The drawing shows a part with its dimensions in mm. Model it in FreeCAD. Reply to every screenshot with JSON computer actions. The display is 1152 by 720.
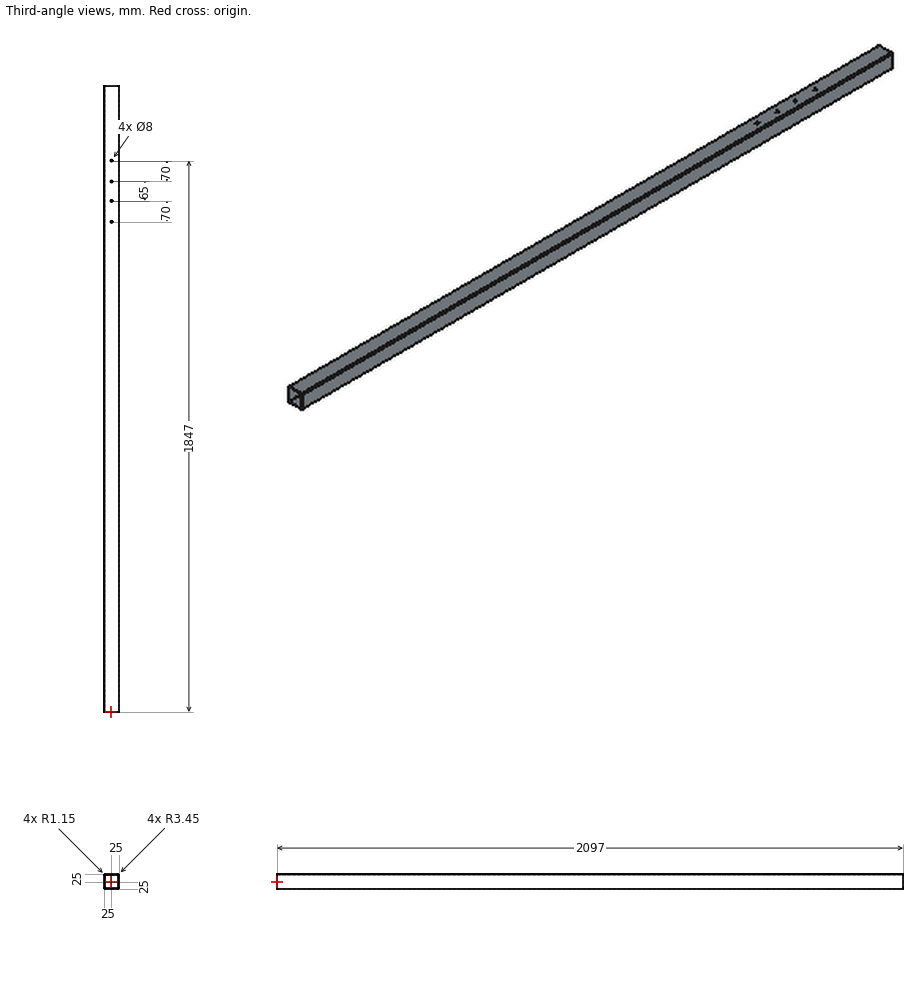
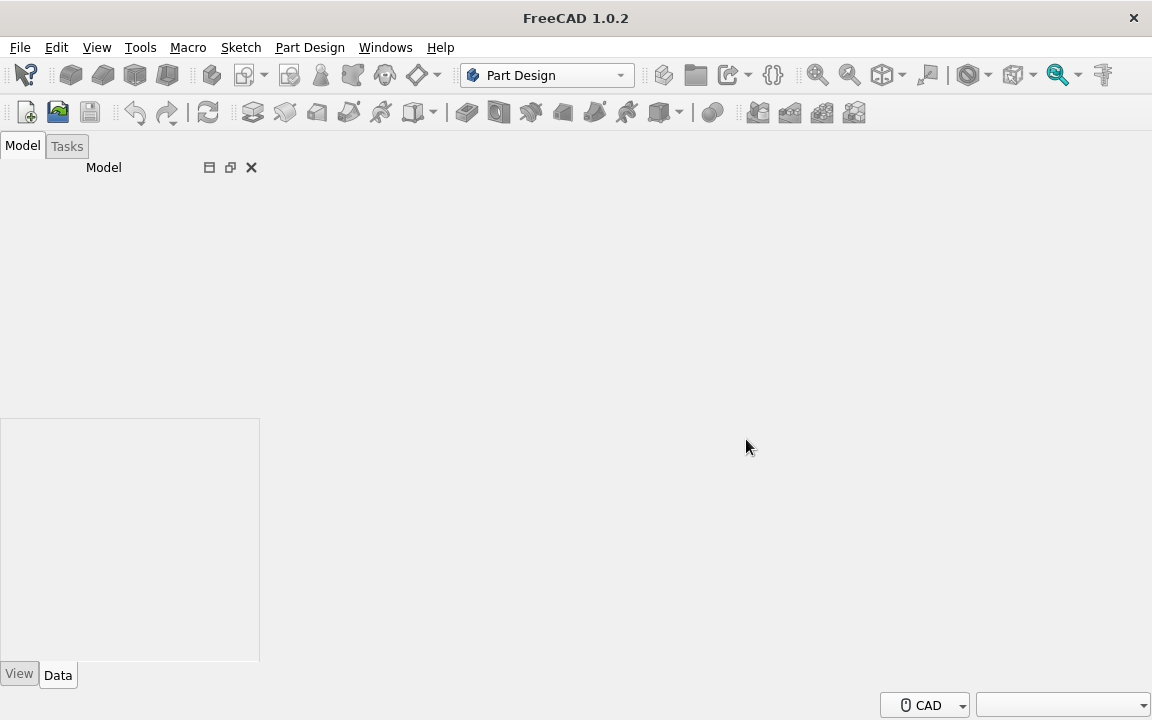
{"action": "left_click", "coordinate": [26, 112]}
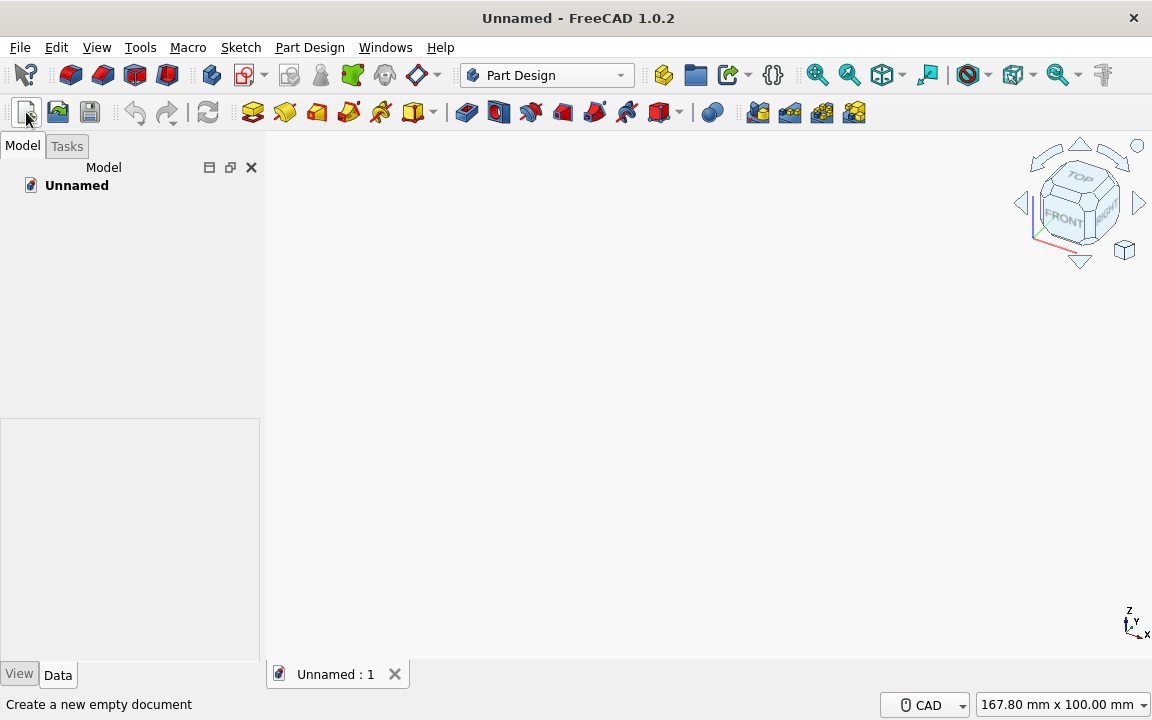
{"action": "left_click", "coordinate": [244, 76]}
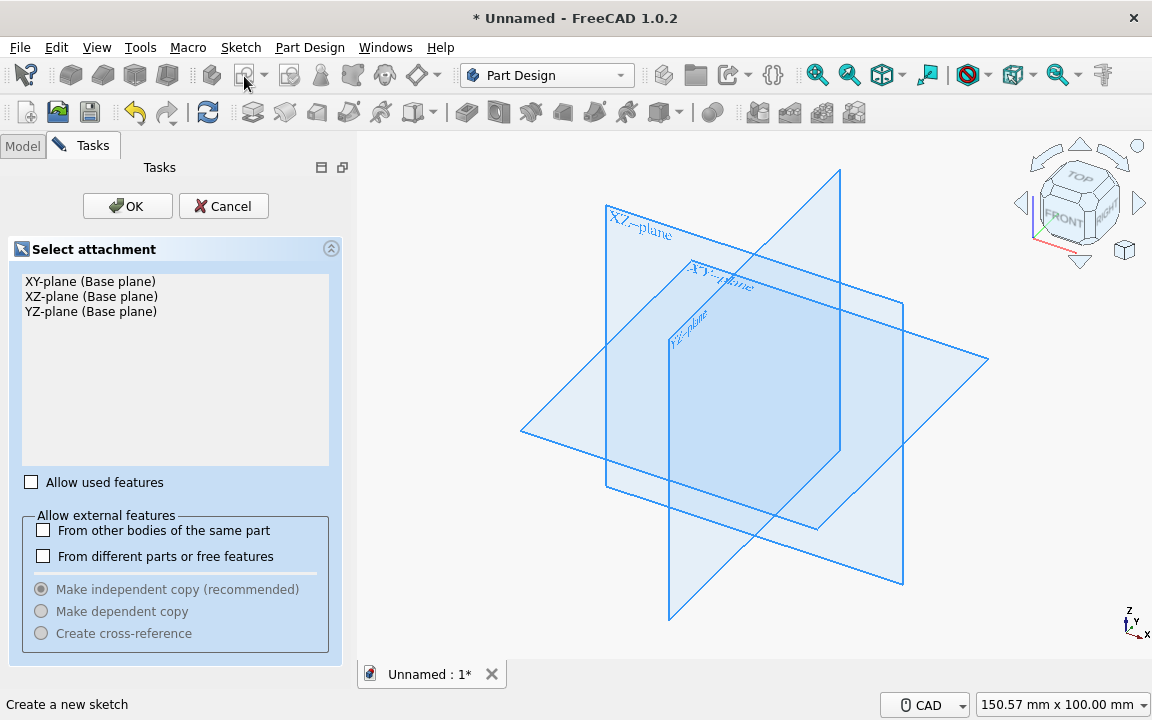
{"action": "left_click", "coordinate": [82, 296]}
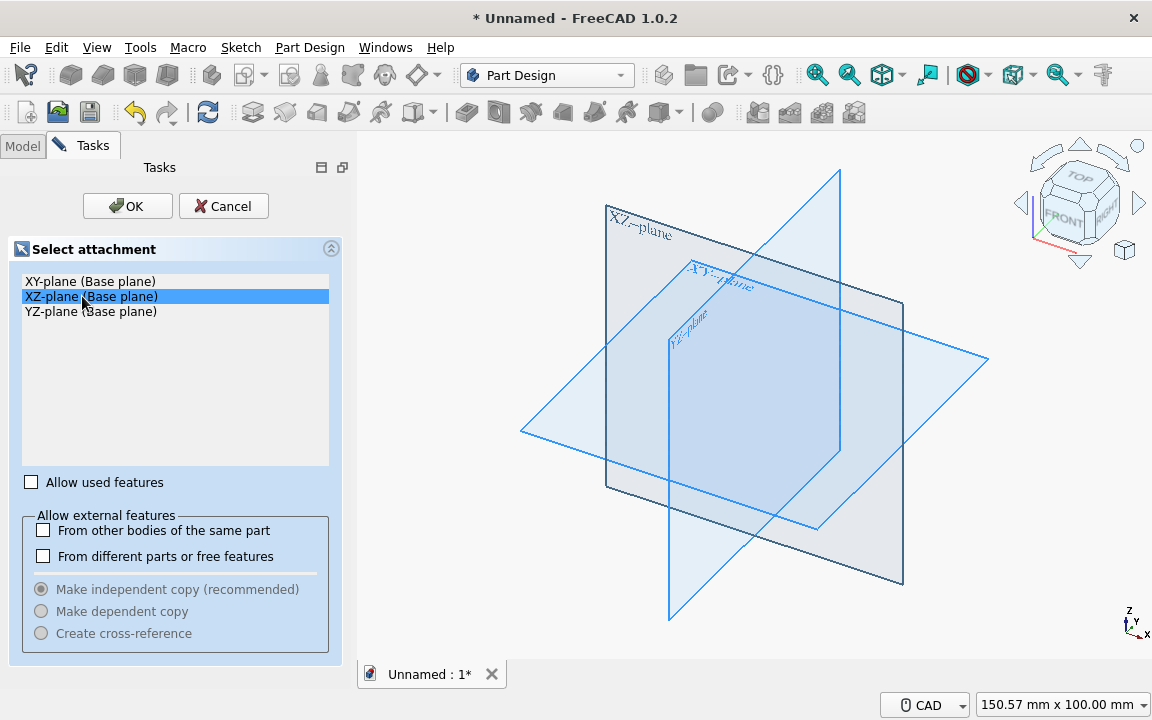
{"action": "left_click", "coordinate": [128, 206]}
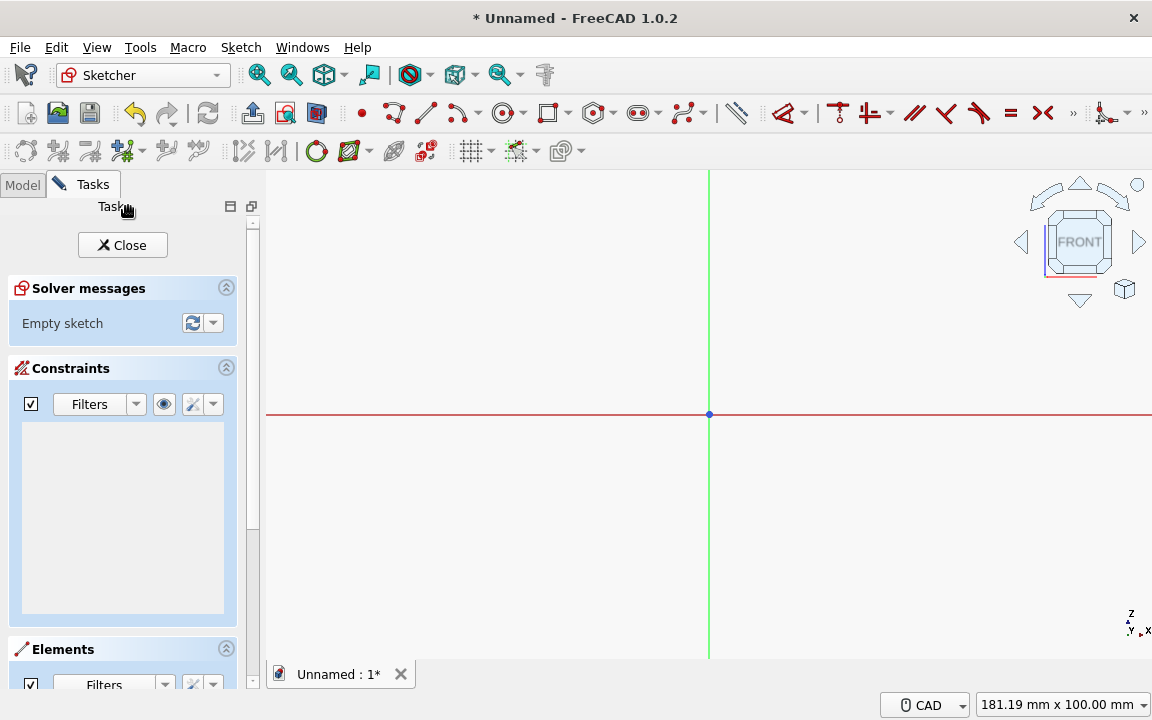
{"action": "left_click", "coordinate": [426, 114]}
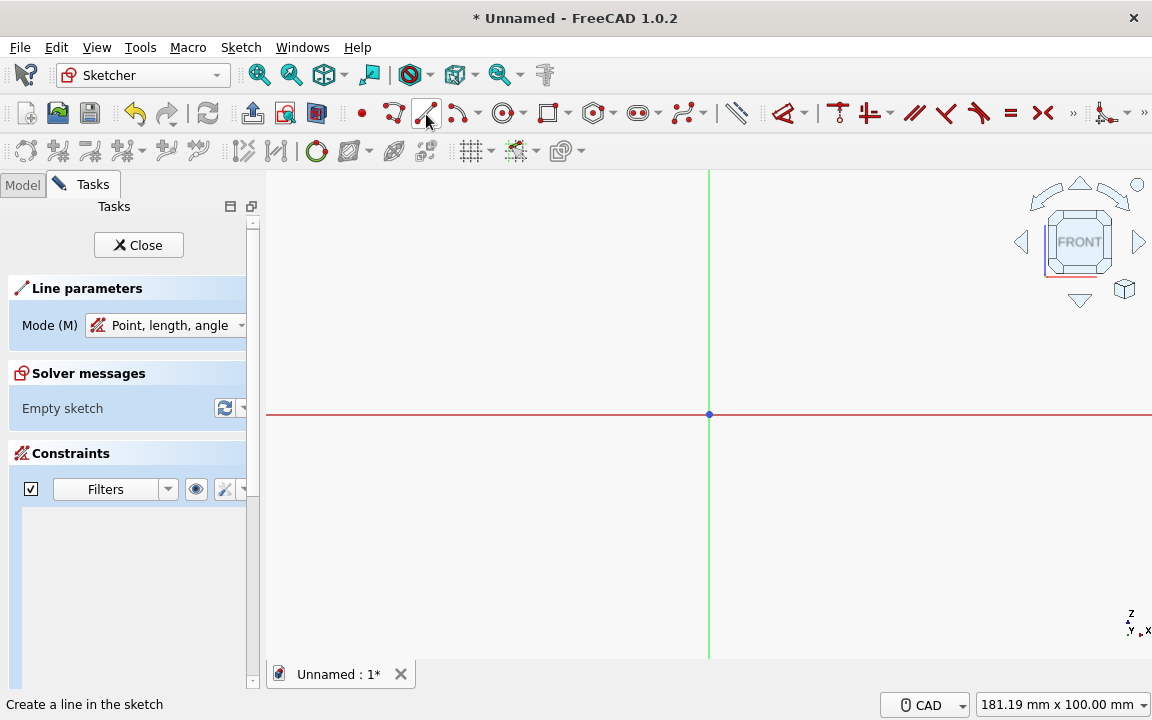
{"action": "left_click", "coordinate": [604, 292]}
{"action": "left_click", "coordinate": [814, 292]}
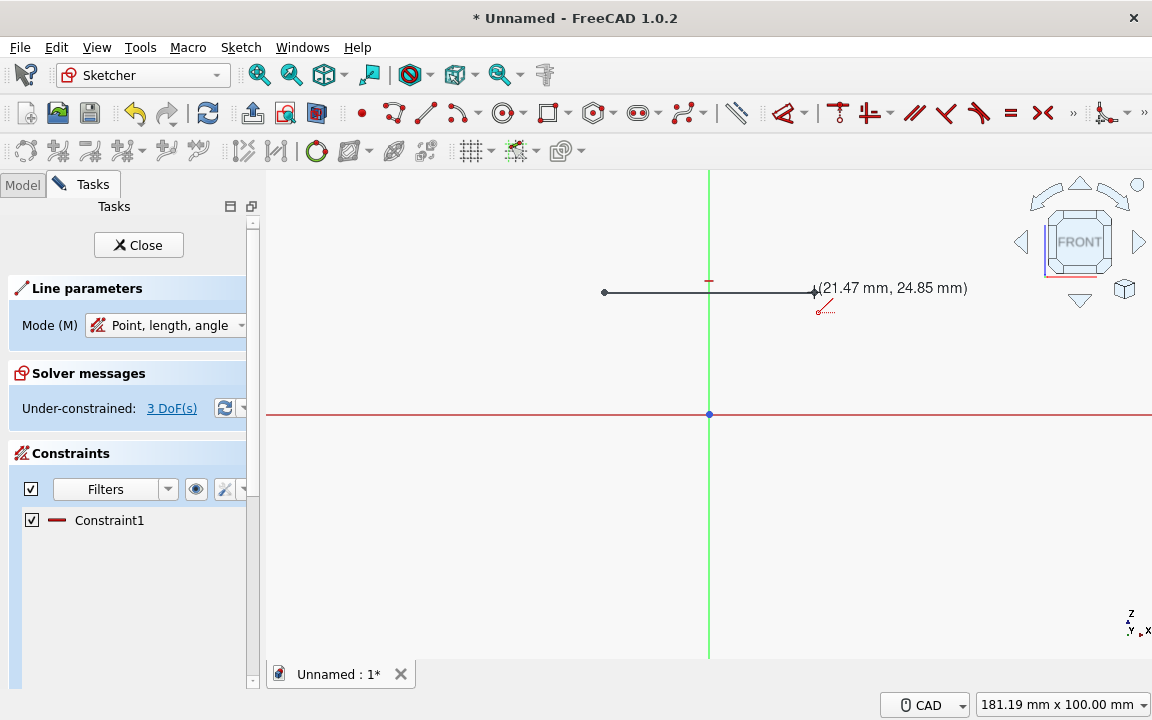
{"action": "left_click", "coordinate": [831, 309]}
{"action": "left_click", "coordinate": [831, 520]}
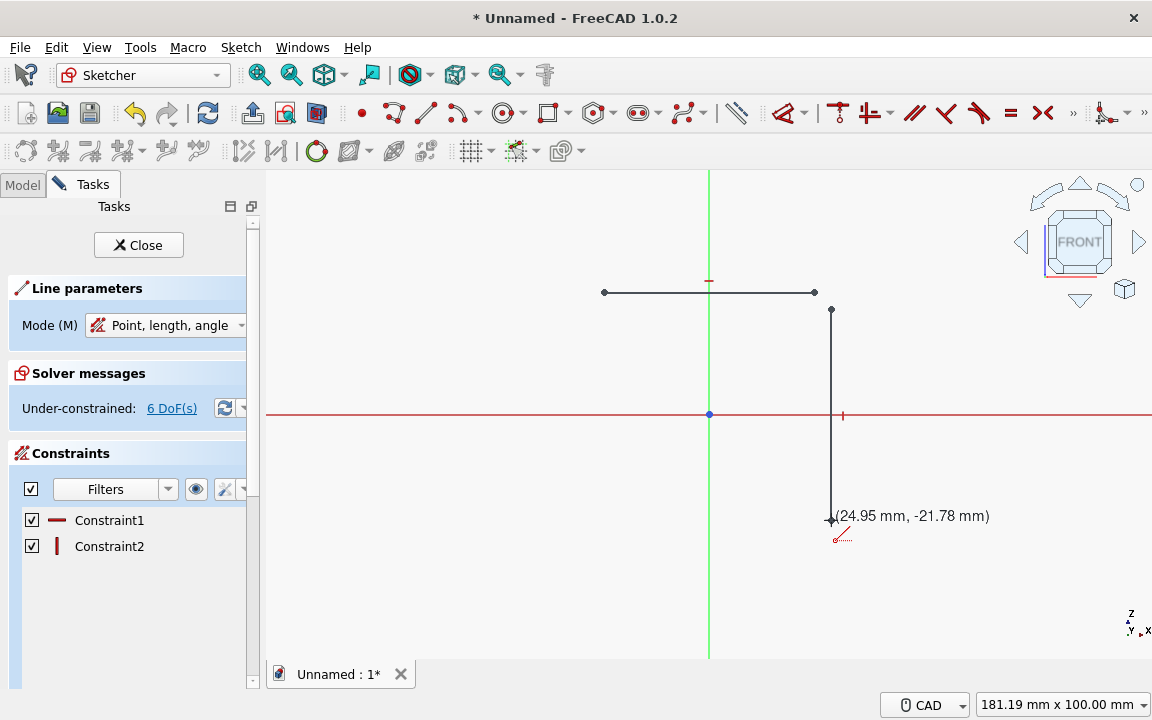
{"action": "left_click", "coordinate": [814, 537]}
{"action": "left_click", "coordinate": [604, 537]}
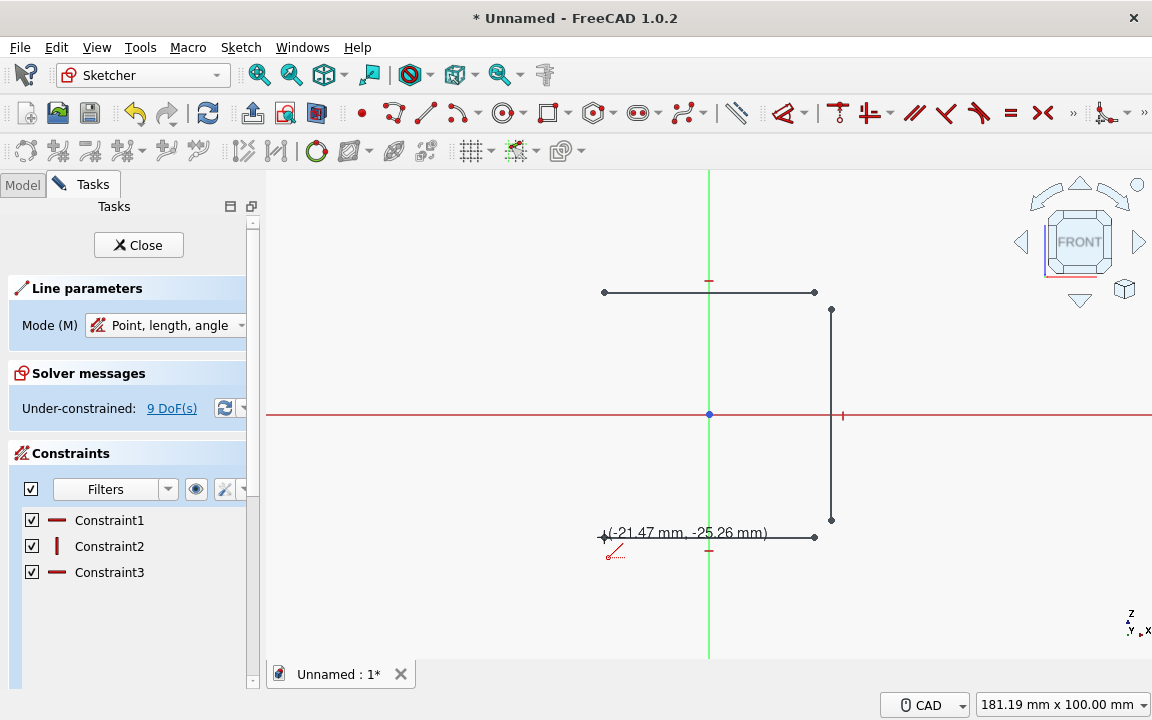
{"action": "left_click", "coordinate": [587, 520]}
{"action": "left_click", "coordinate": [587, 309]}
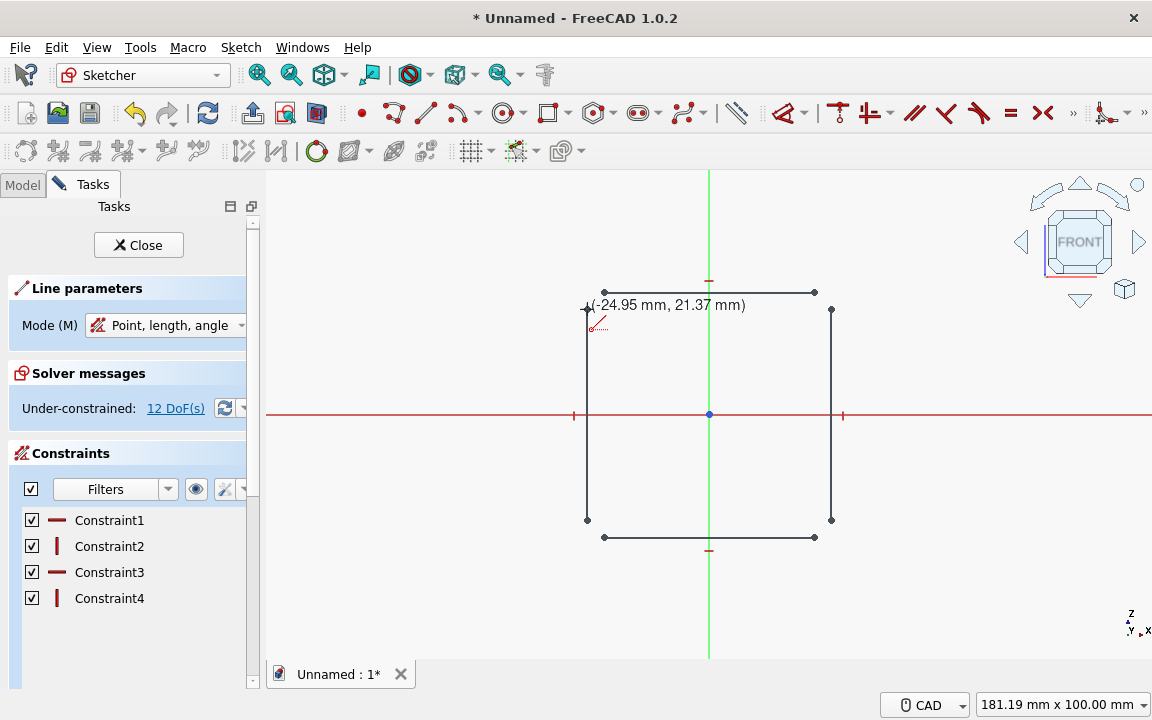
{"action": "key", "text": "g 3 a"}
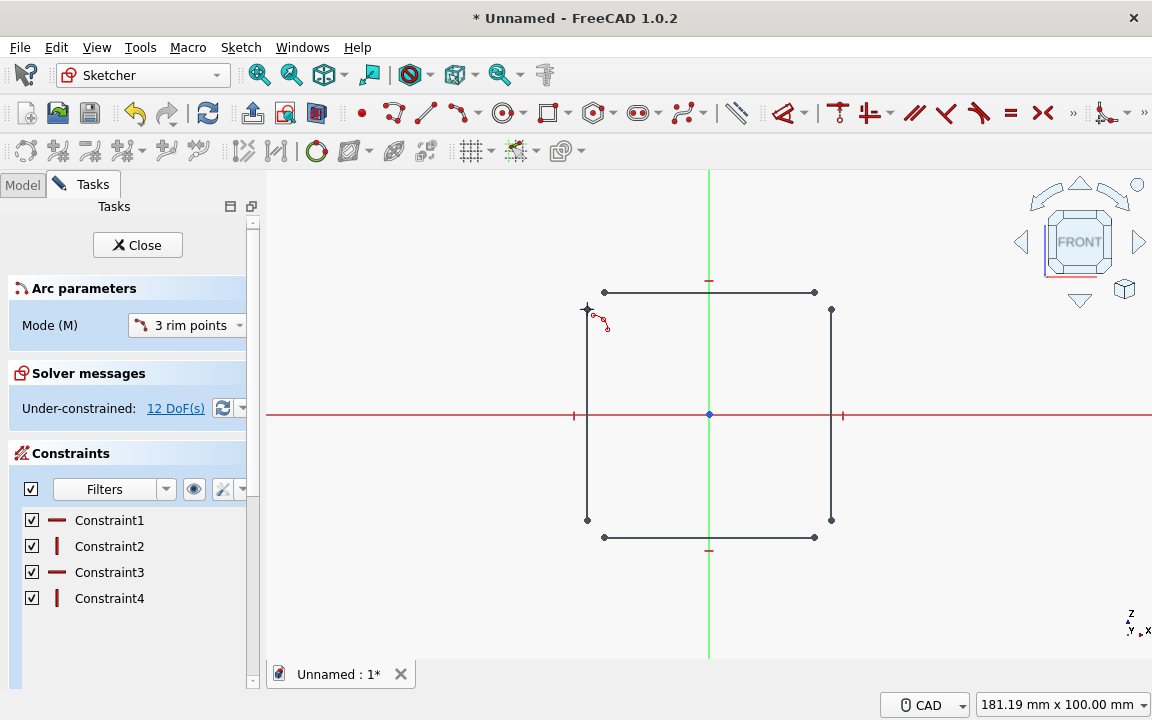
{"action": "left_click", "coordinate": [814, 293]}
{"action": "left_click", "coordinate": [831, 310]}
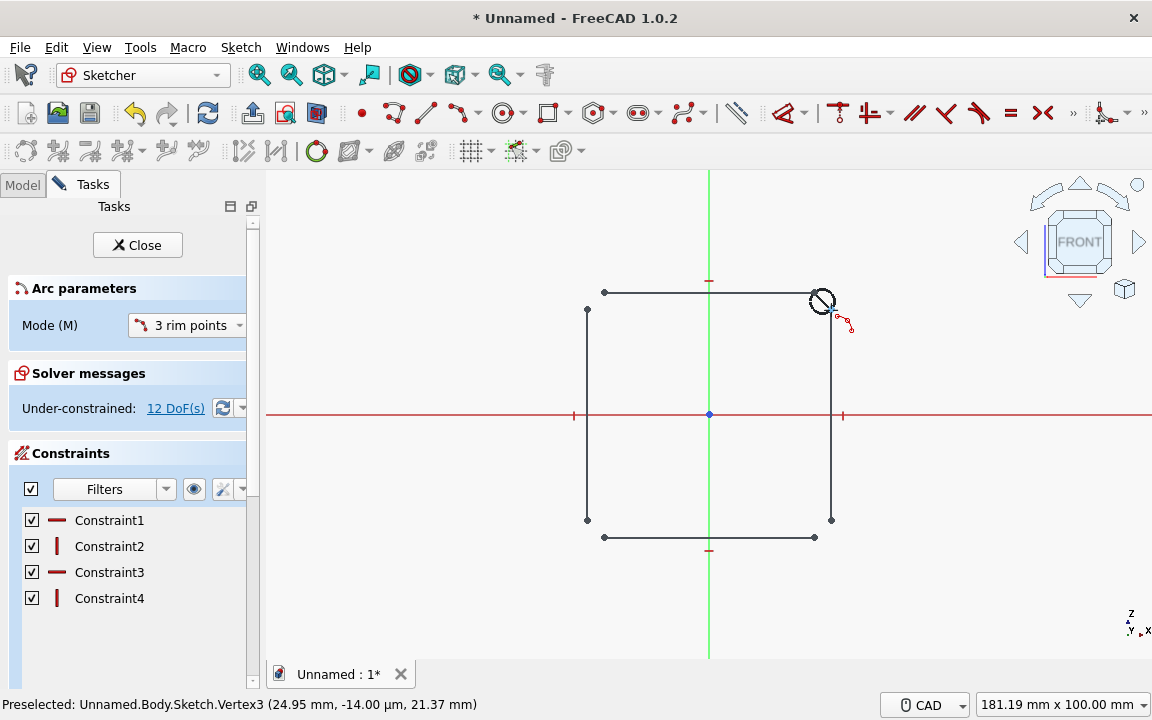
{"action": "scroll", "coordinate": [826, 297], "scroll_direction": "up", "scroll_amount": 6}